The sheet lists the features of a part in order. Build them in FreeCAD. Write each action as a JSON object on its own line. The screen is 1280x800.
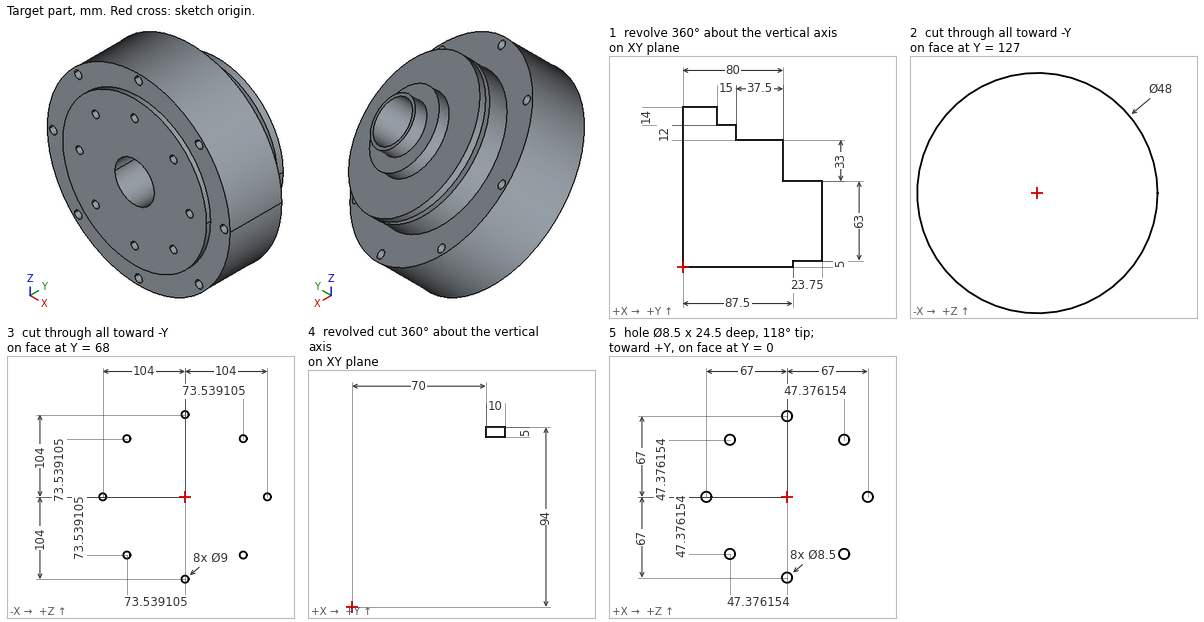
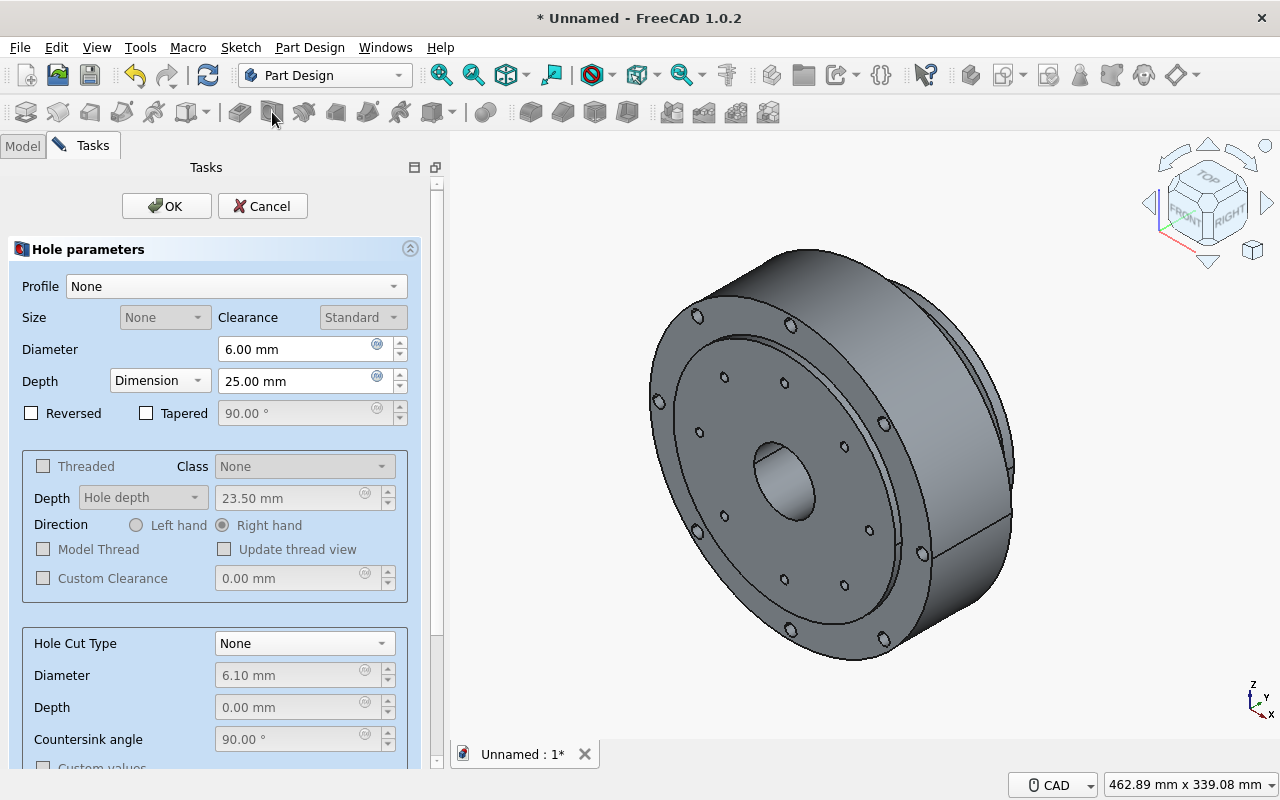
{"action": "triple_click", "coordinate": [305, 349]}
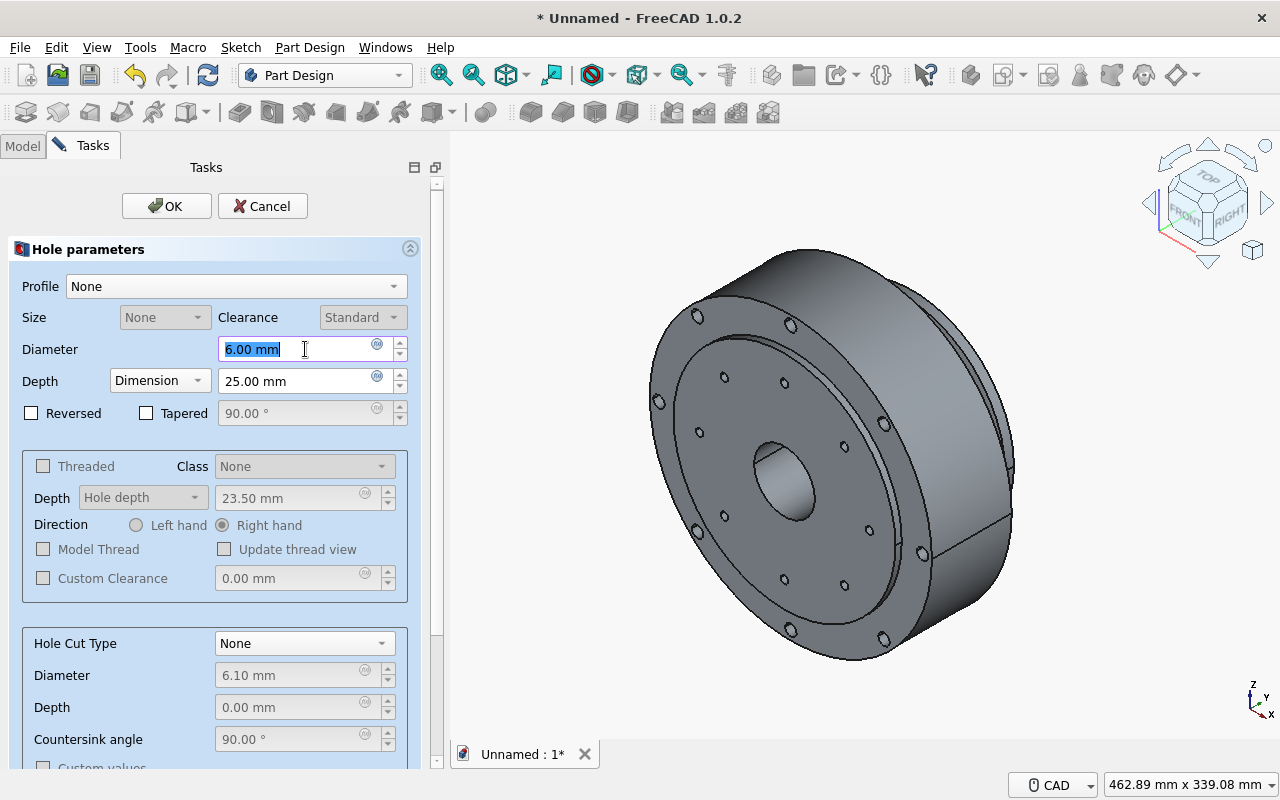
{"action": "type", "text": "8.5"}
{"action": "key", "text": "Tab"}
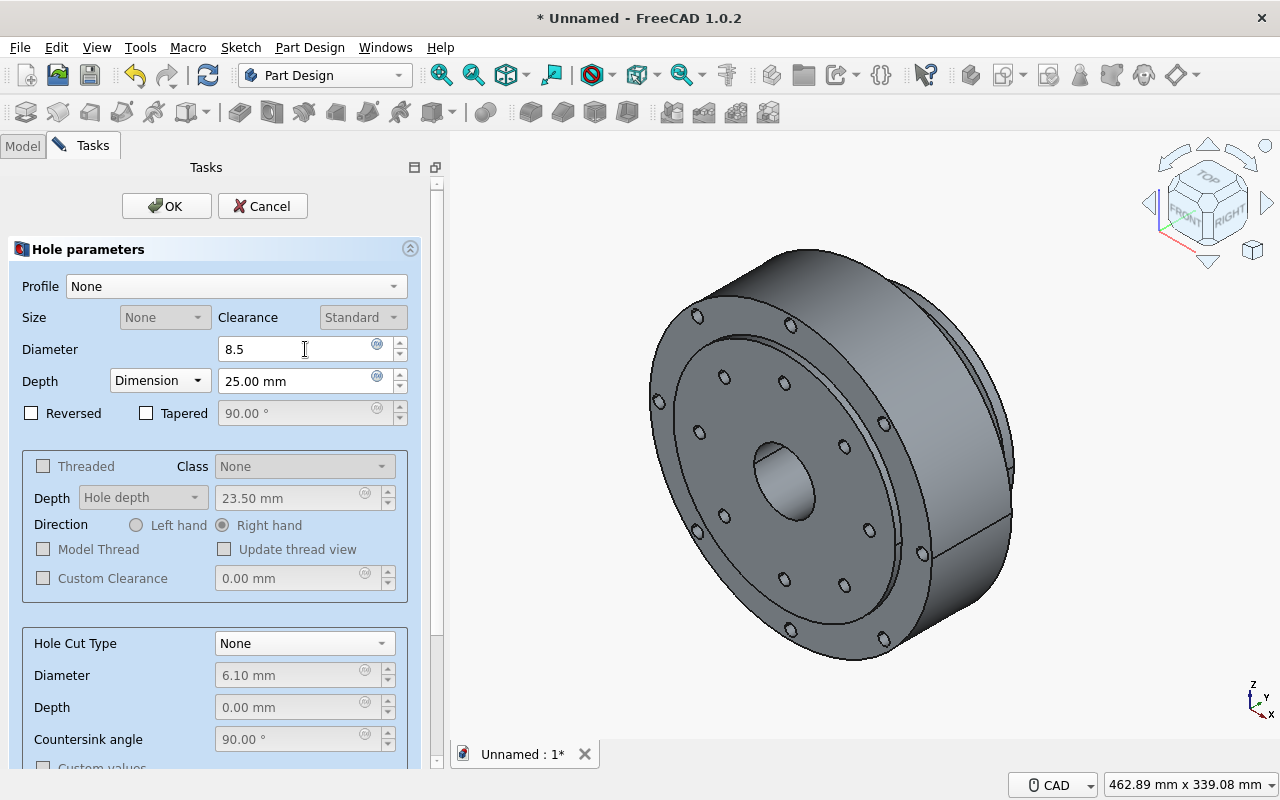
{"action": "triple_click", "coordinate": [305, 381]}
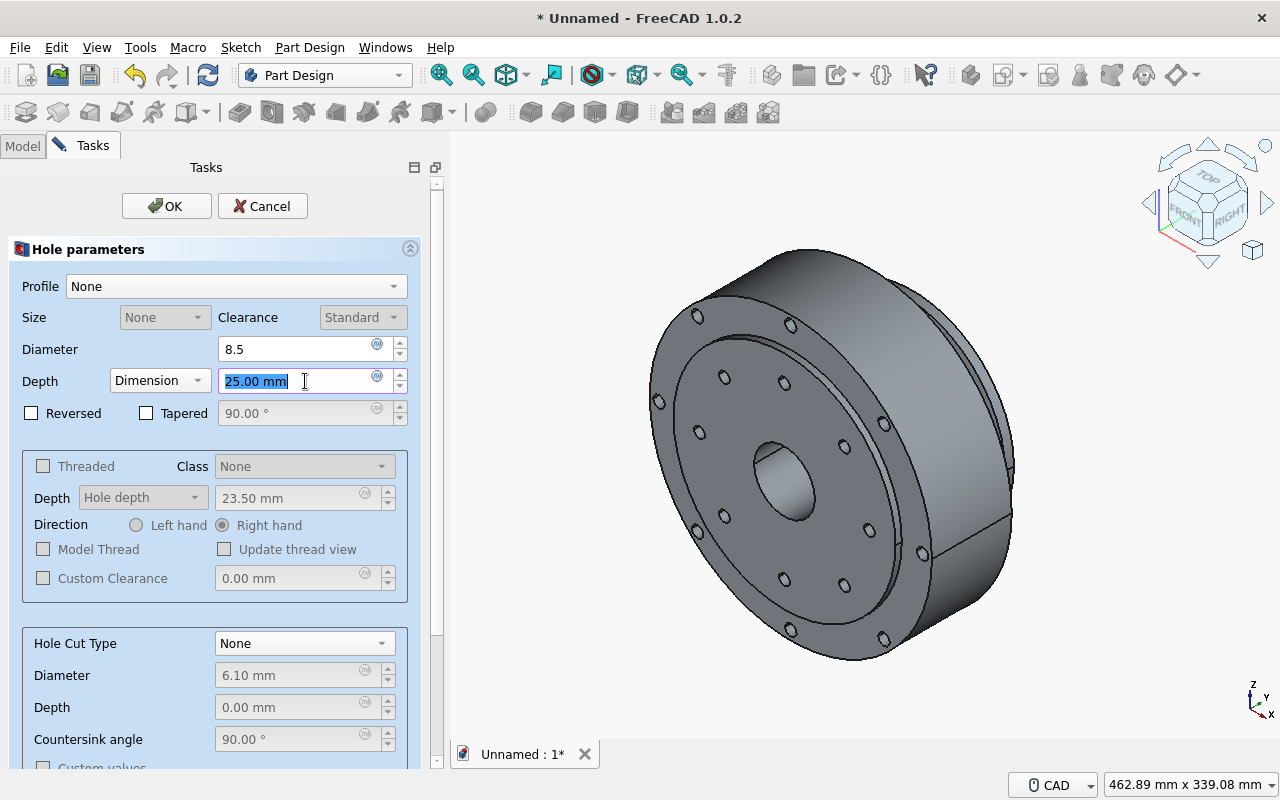
{"action": "type", "text": "24.5"}
{"action": "key", "text": "Tab"}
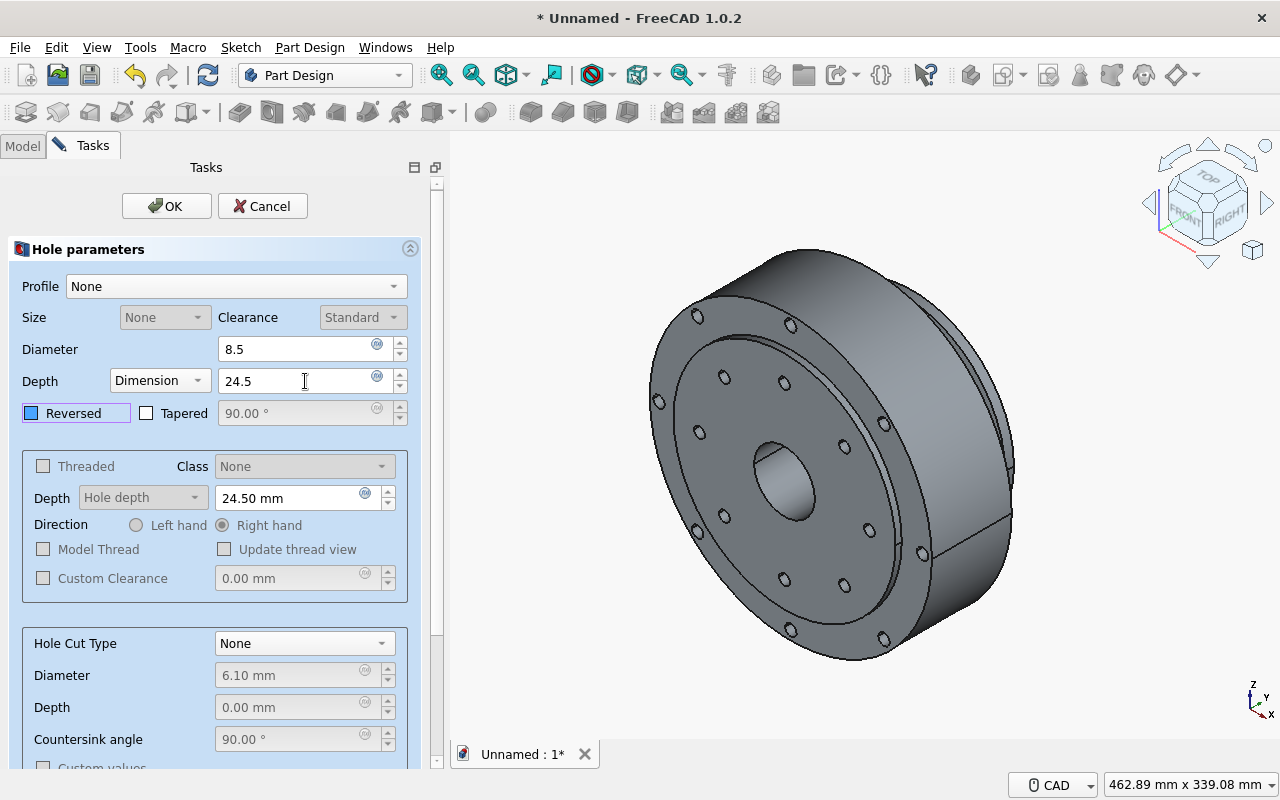
{"action": "left_click", "coordinate": [167, 206]}